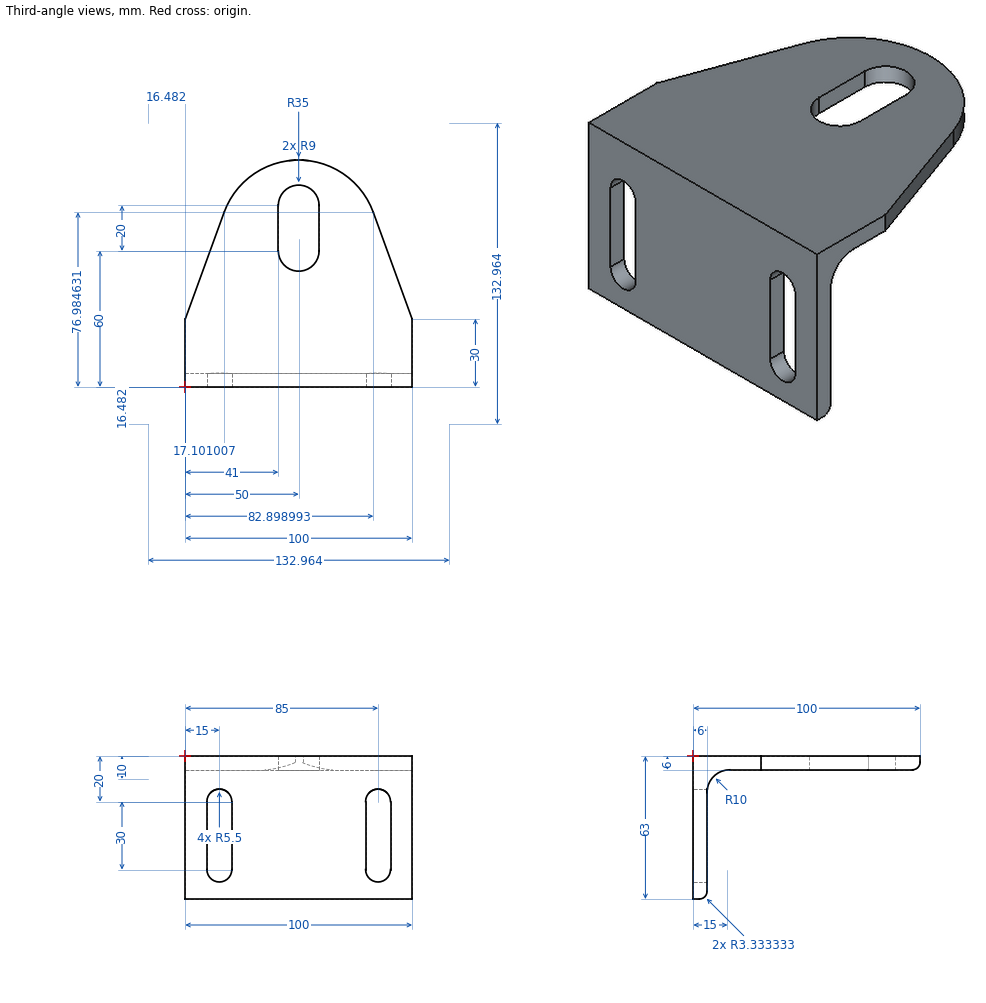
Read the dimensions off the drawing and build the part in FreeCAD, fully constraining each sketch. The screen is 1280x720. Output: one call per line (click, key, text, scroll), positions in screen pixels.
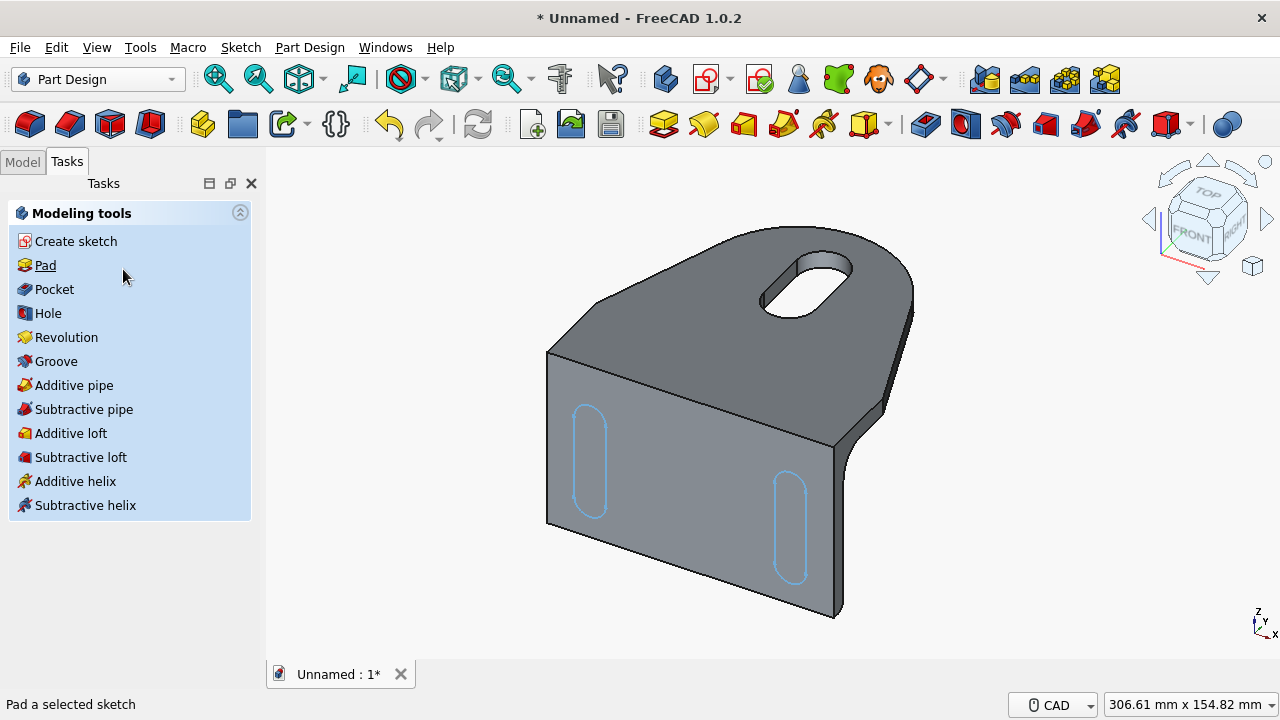
click(926, 124)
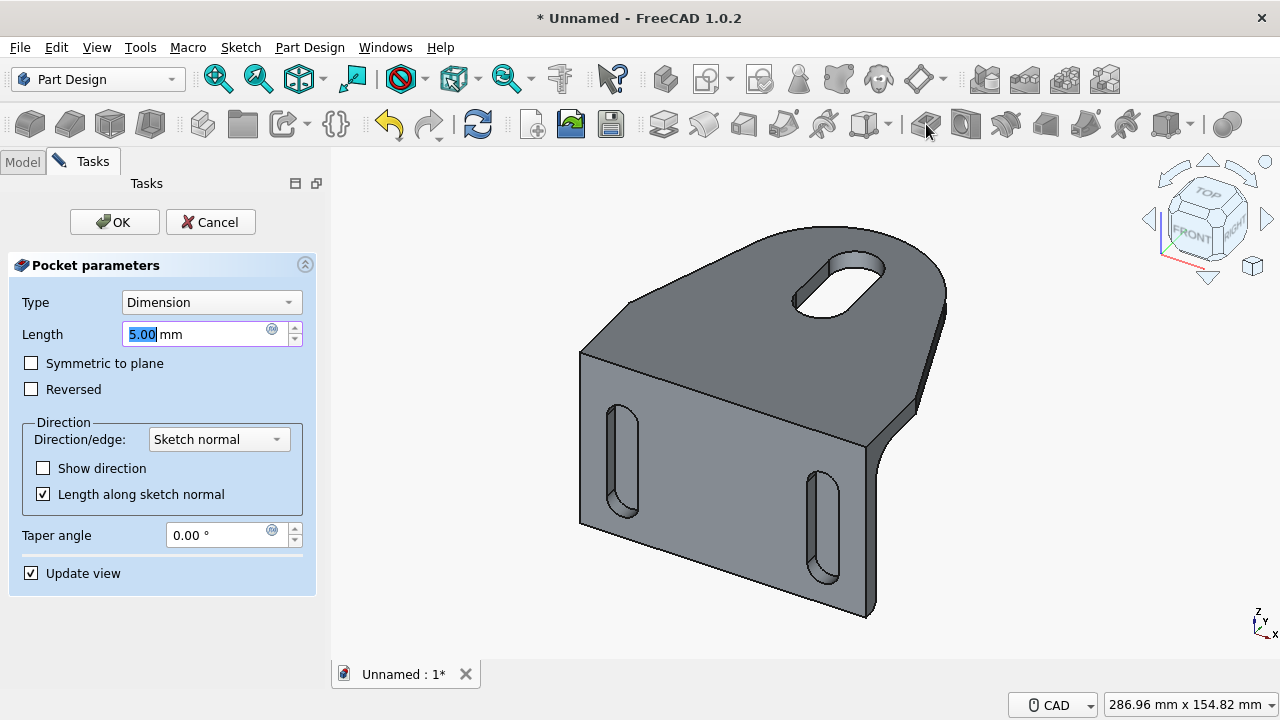
text(15)
key(Tab)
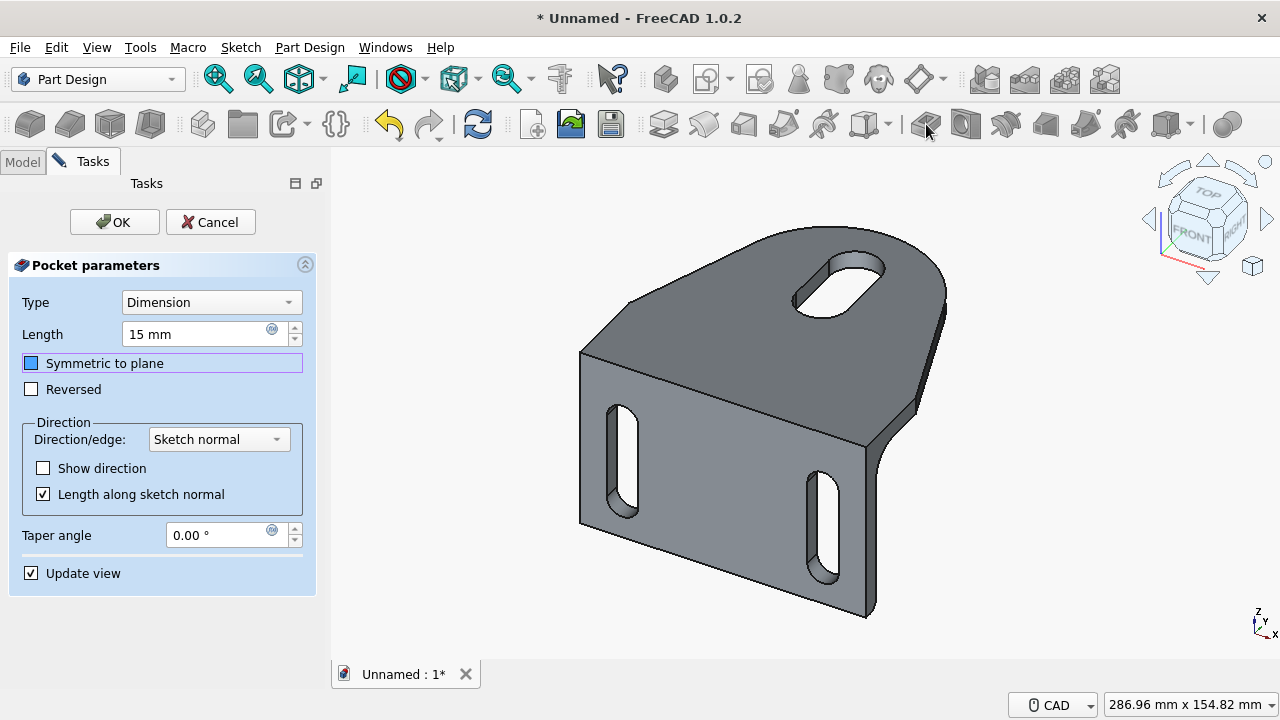
click(115, 222)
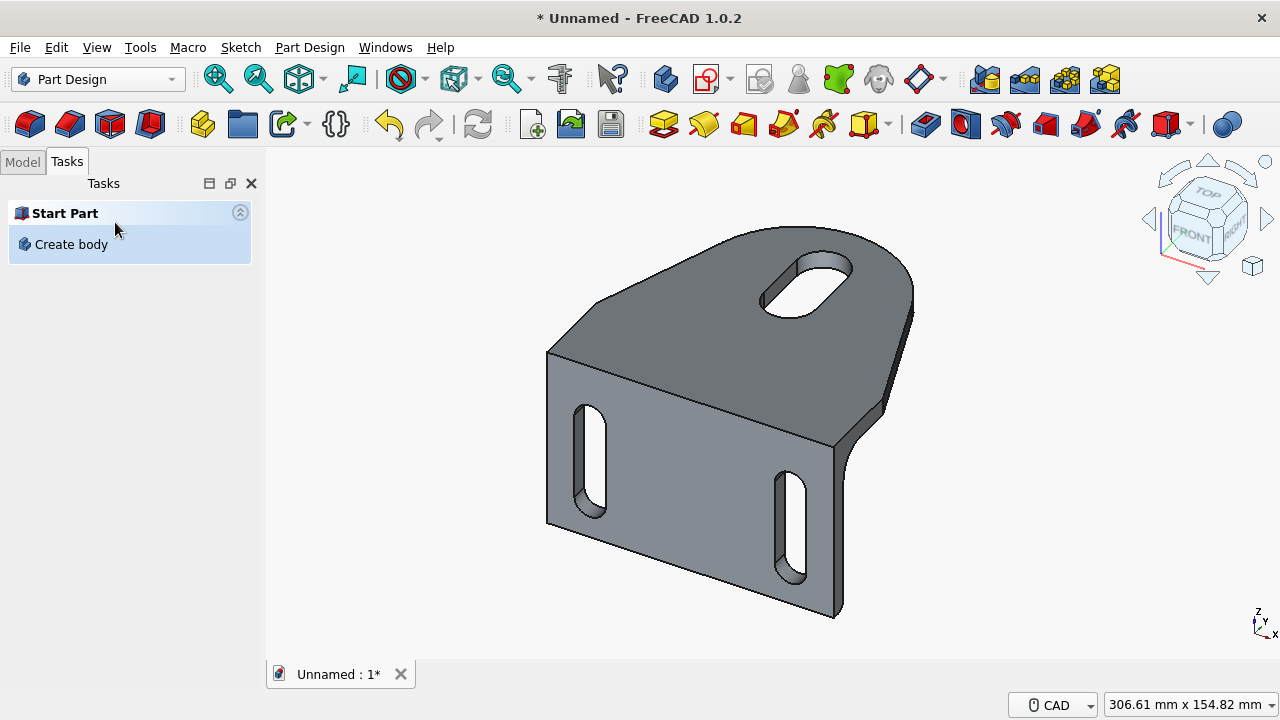
key(0)